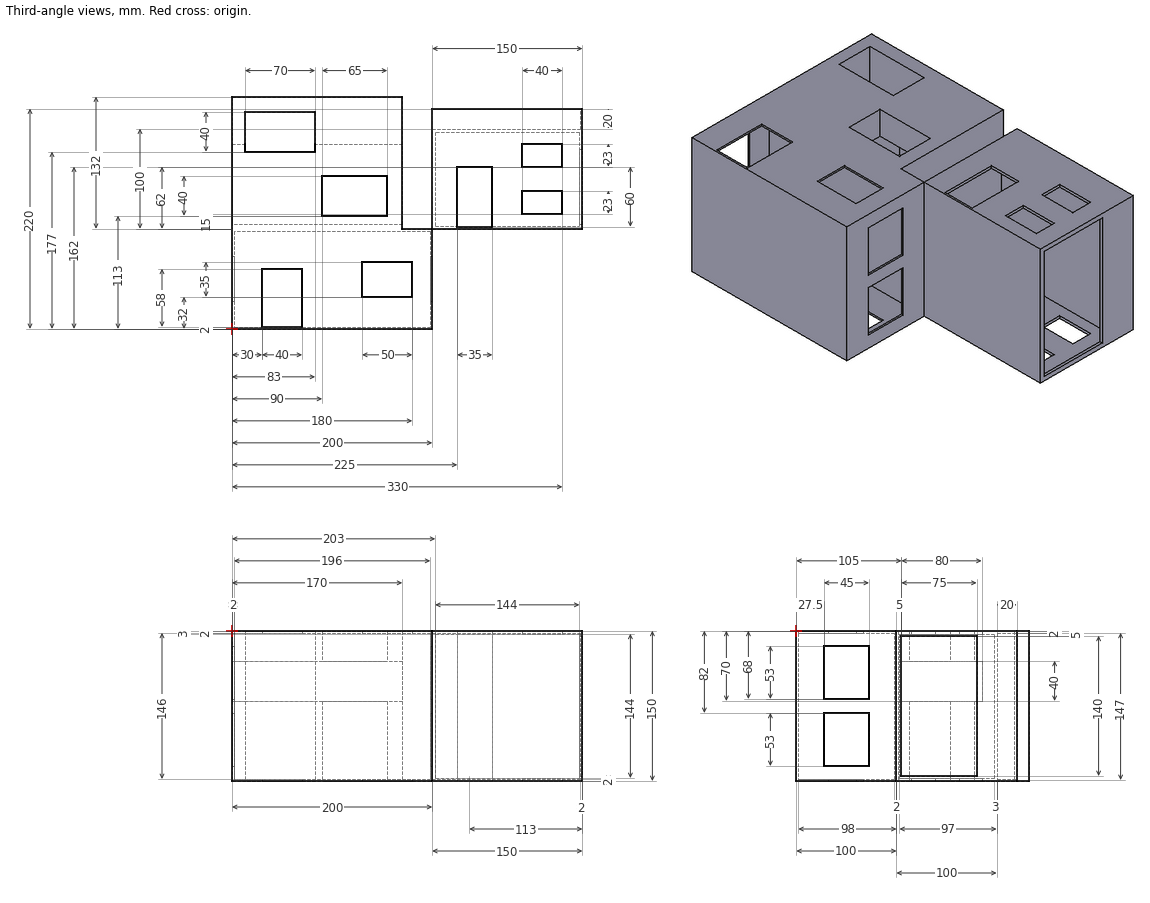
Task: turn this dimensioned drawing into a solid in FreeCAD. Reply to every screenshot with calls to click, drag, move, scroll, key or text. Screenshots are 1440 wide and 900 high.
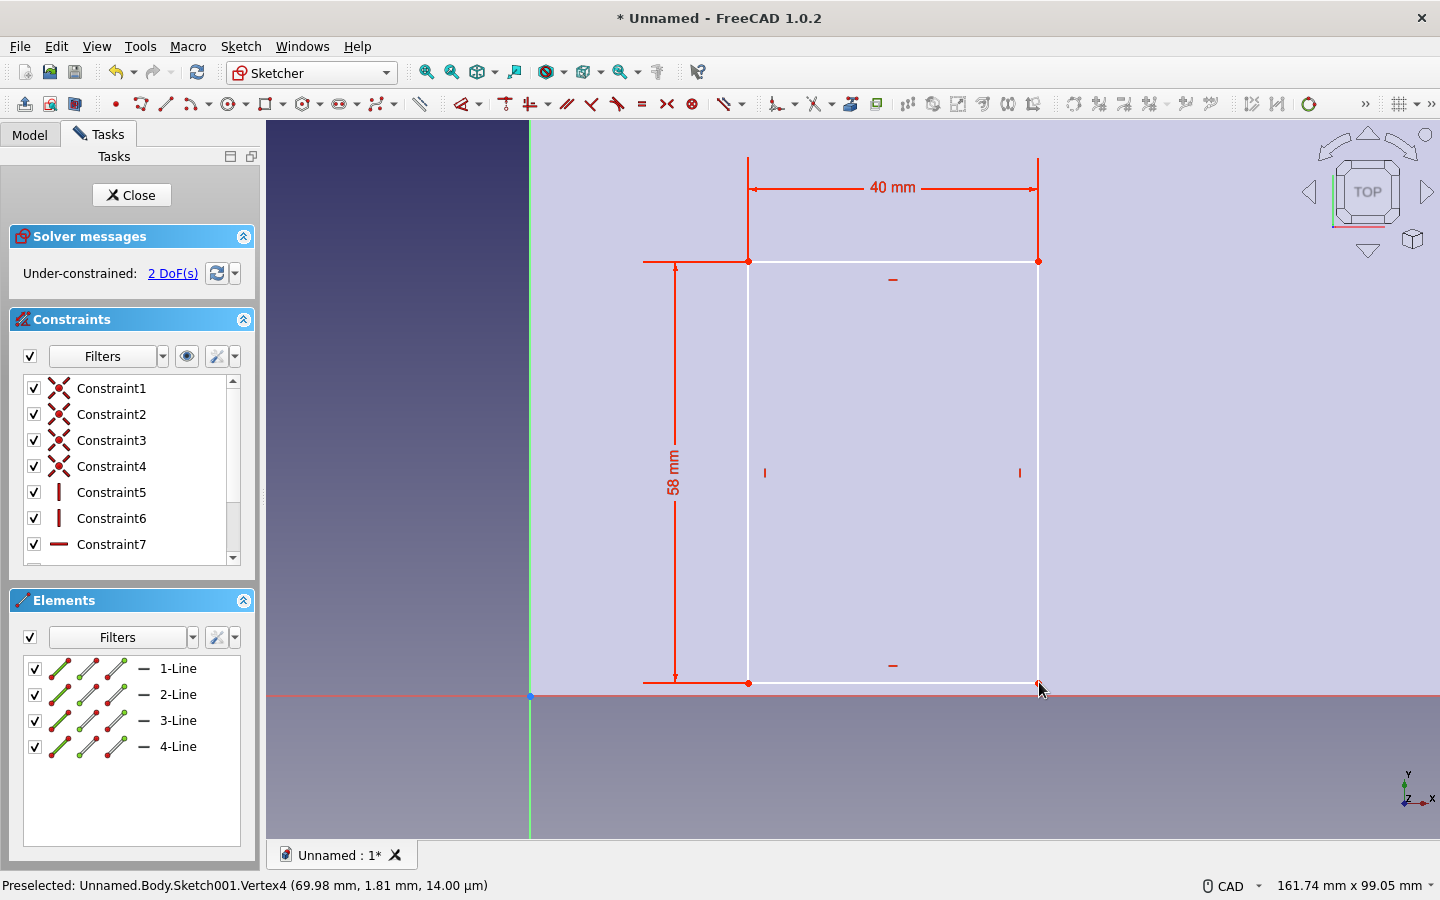
click(460, 104)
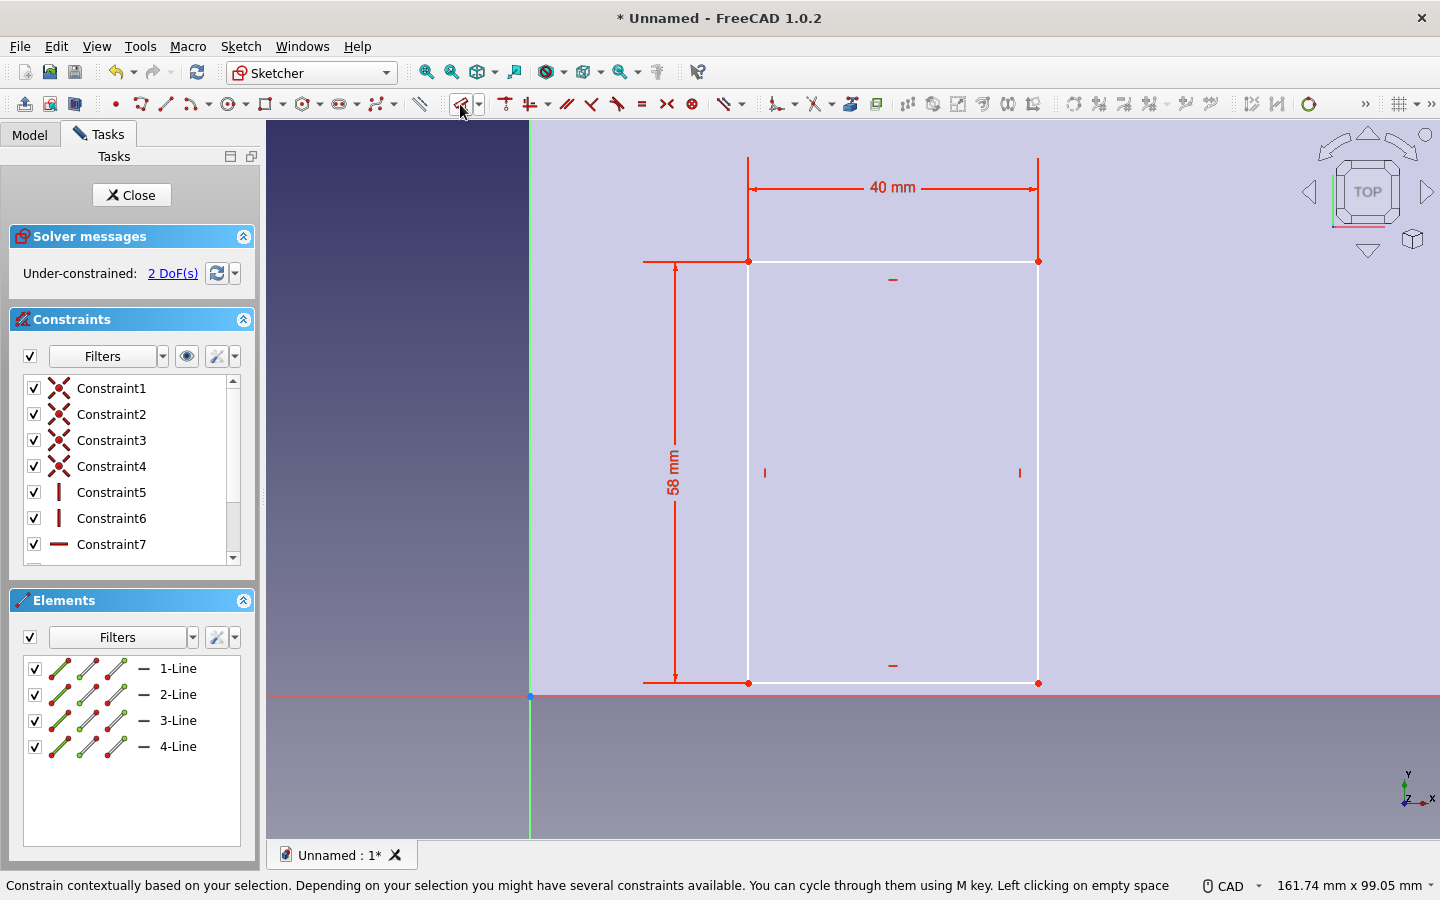
scroll(748, 683, up, 6)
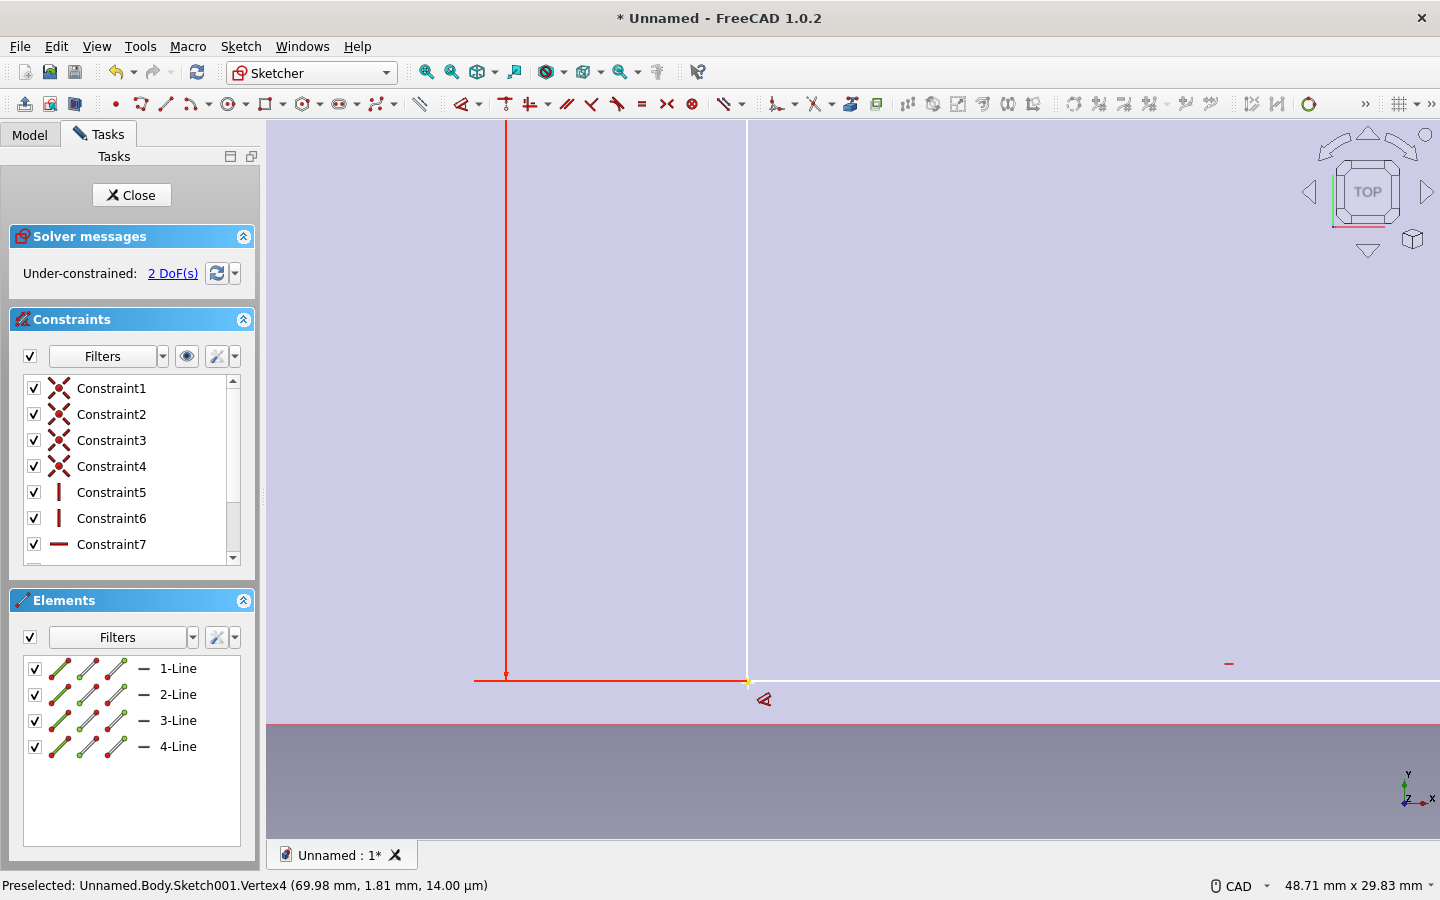
click(747, 681)
click(781, 703)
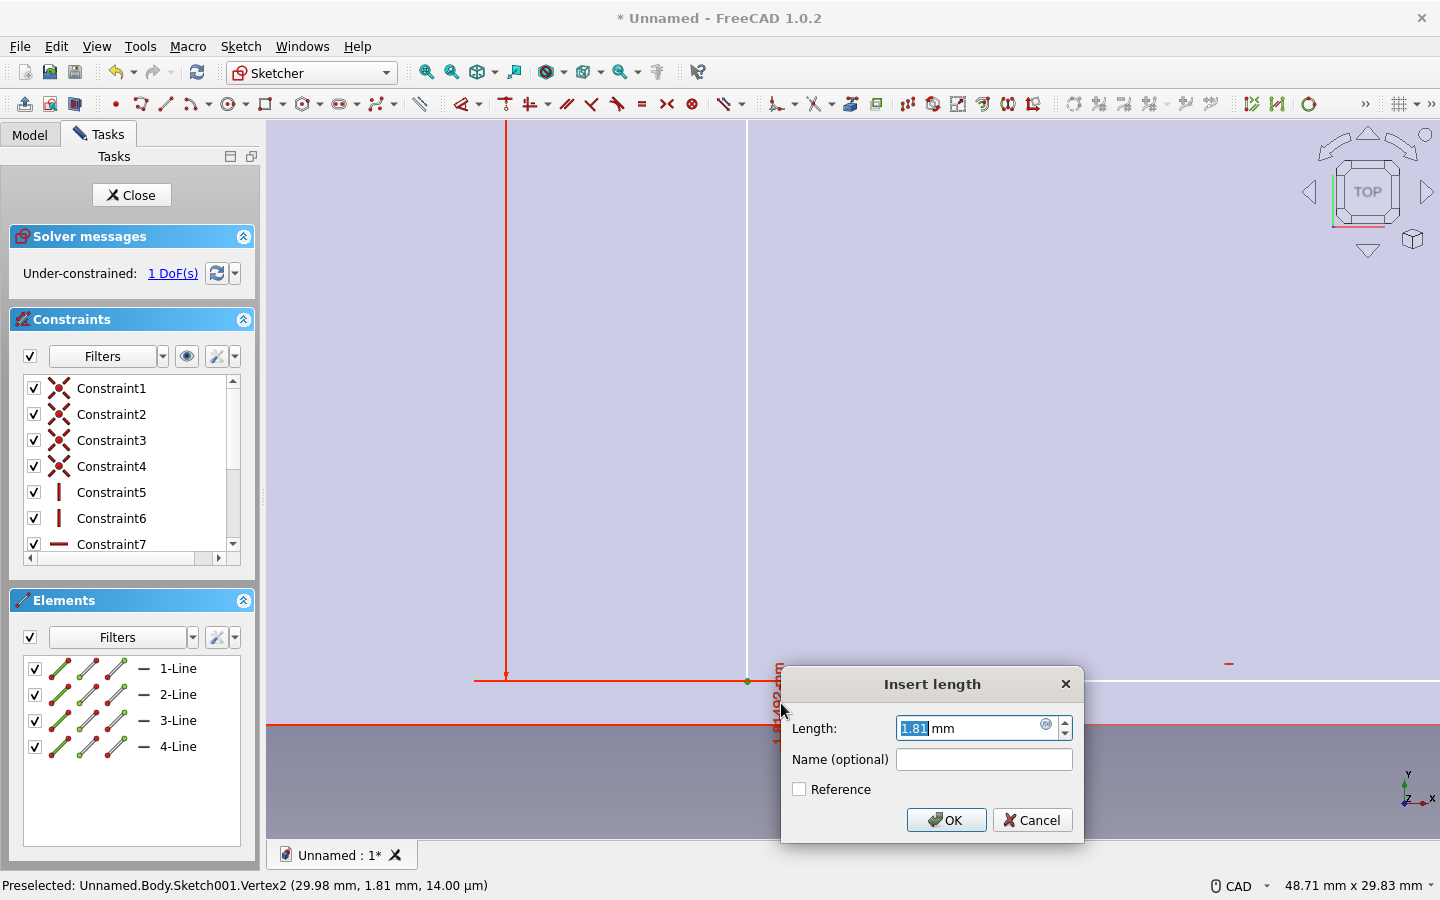
text(2)
key(Return)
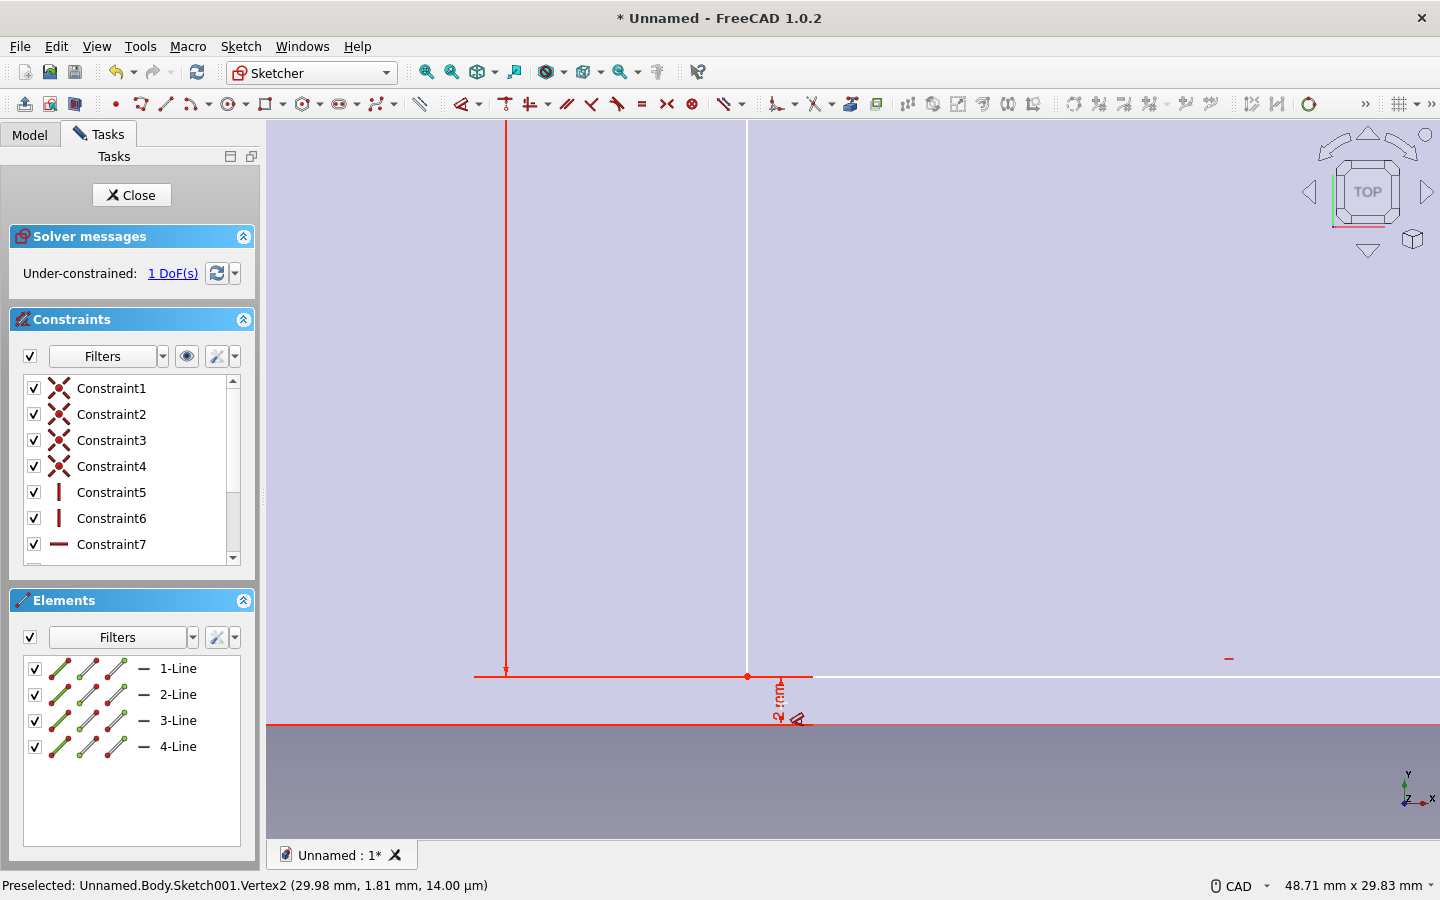
scroll(748, 685, down, 6)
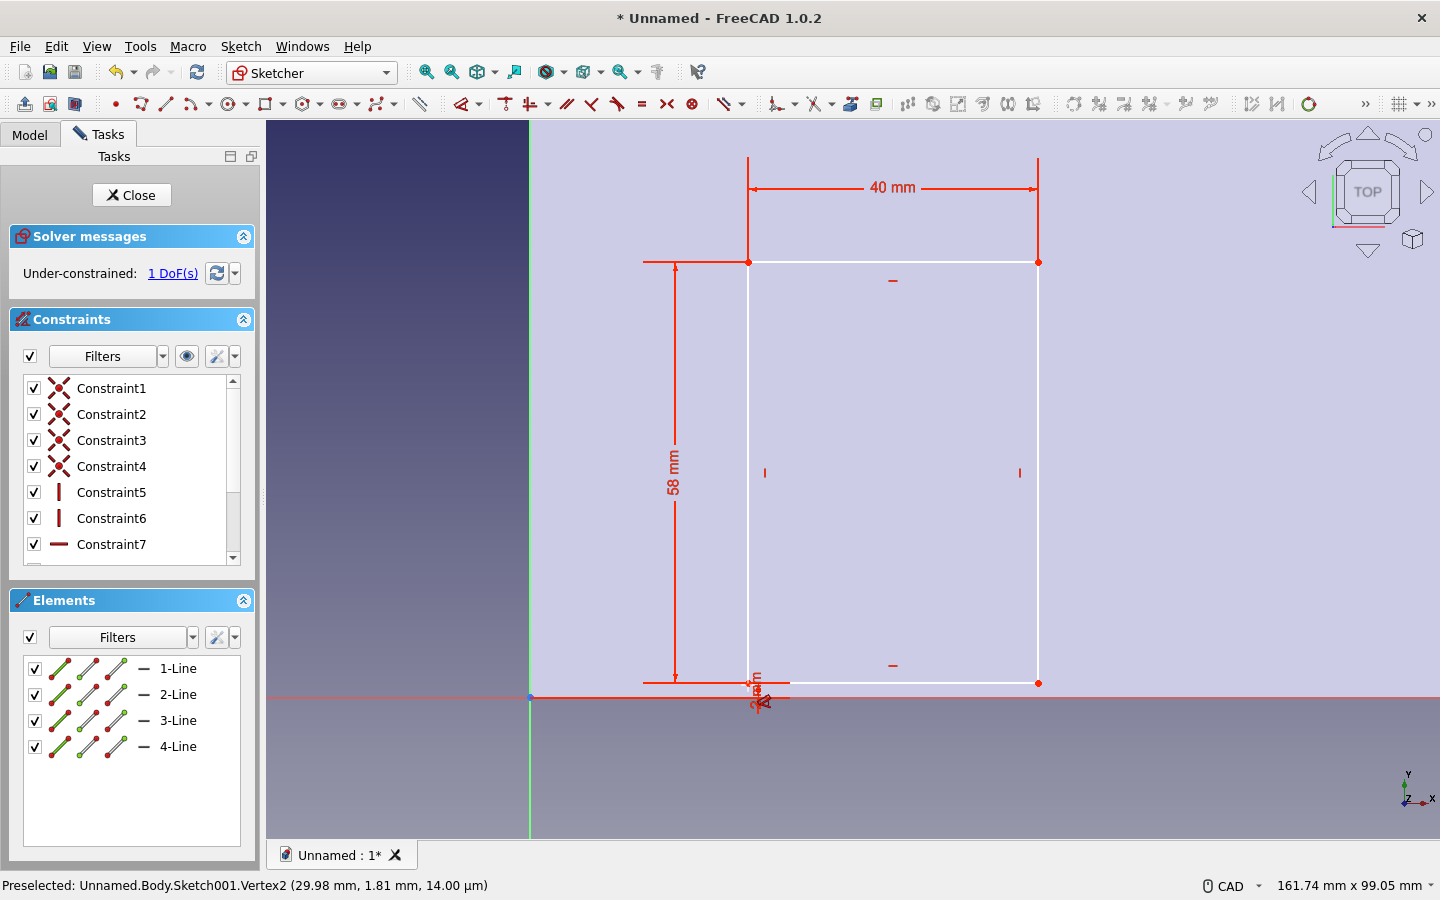
click(748, 262)
click(639, 732)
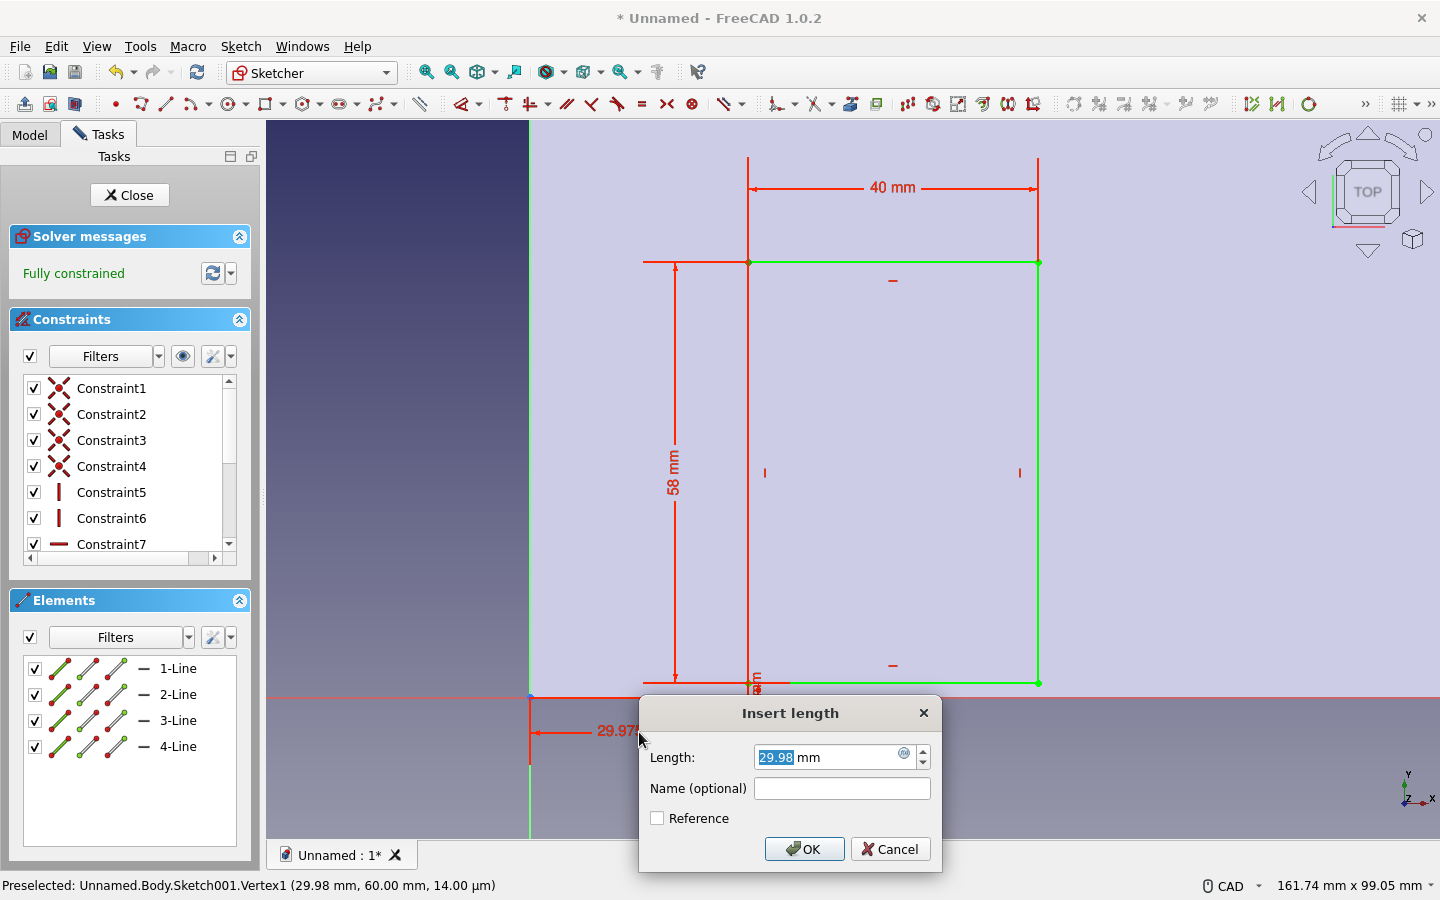
text(30)
key(Return)
key(Escape)